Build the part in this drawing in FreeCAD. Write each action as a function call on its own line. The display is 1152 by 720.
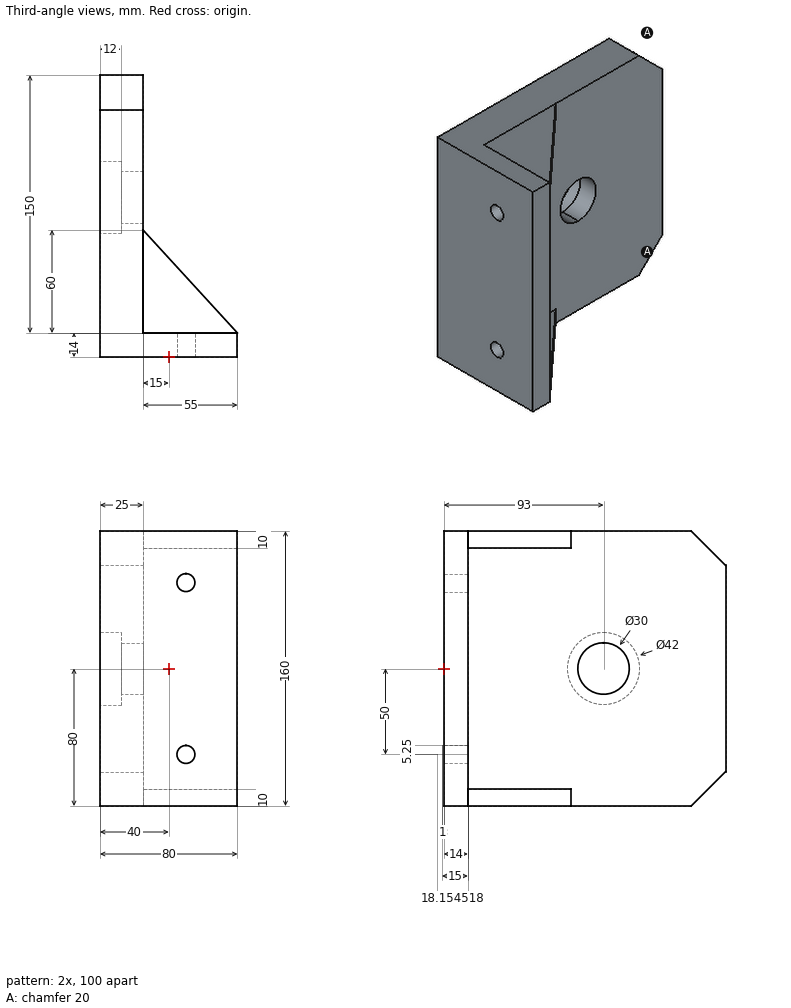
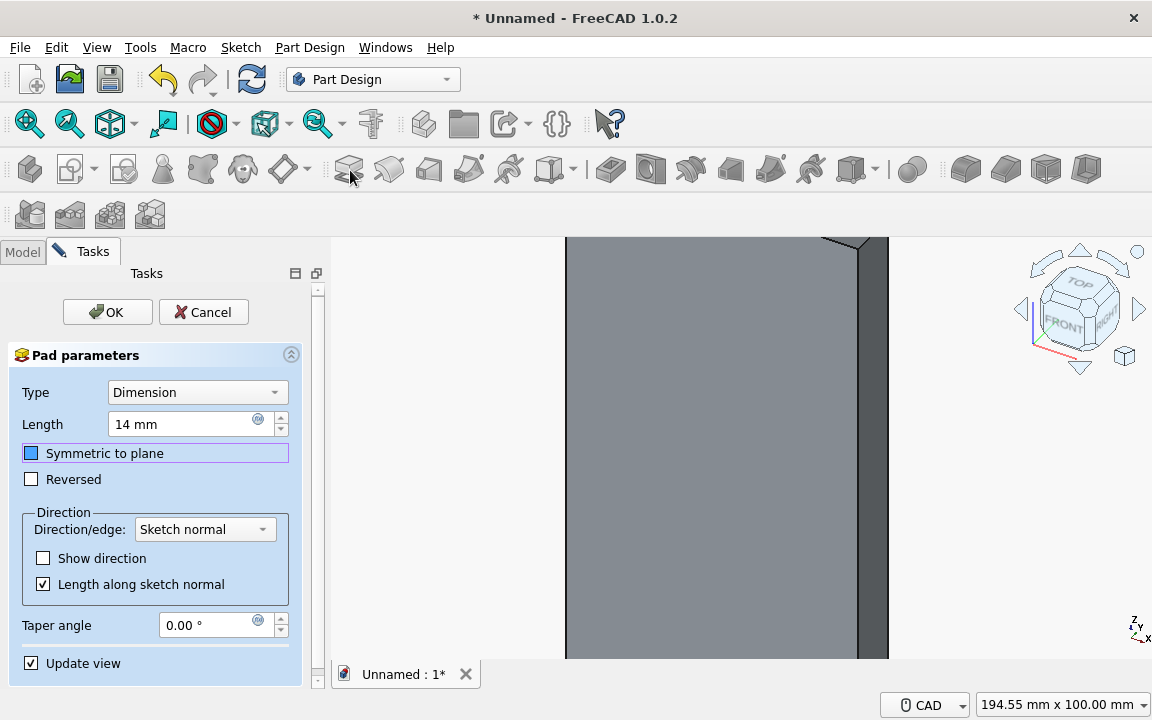
click(30, 479)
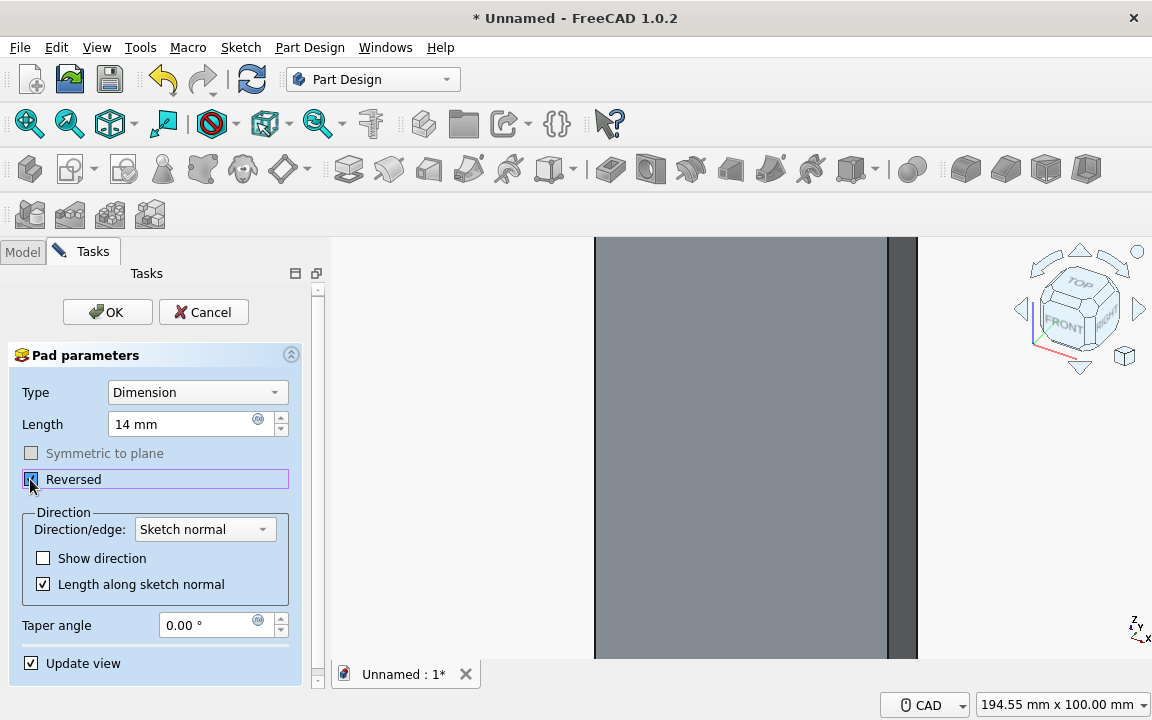
click(108, 312)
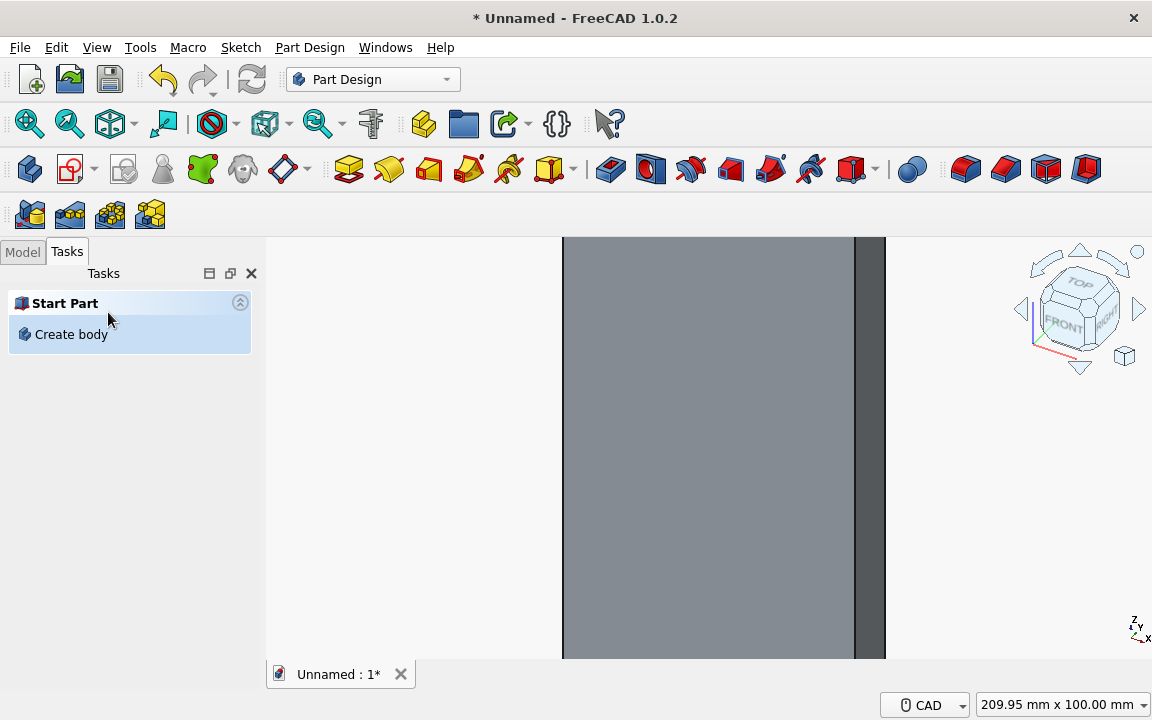
key(v)
key(f)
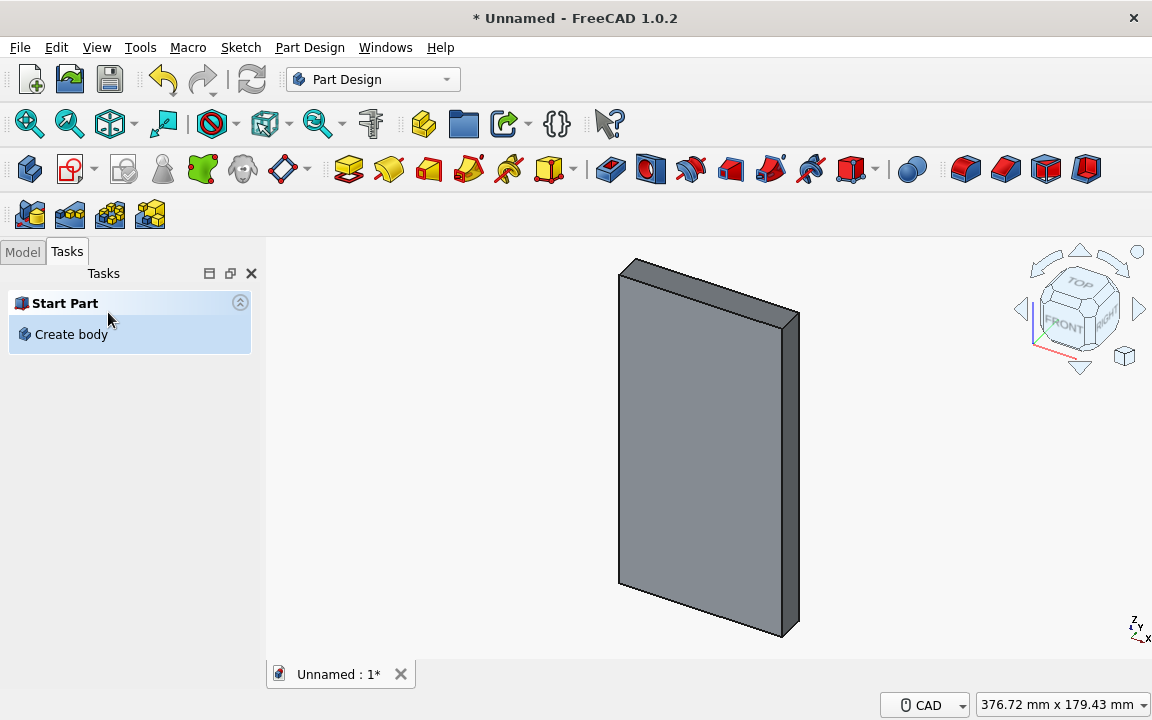
key(4)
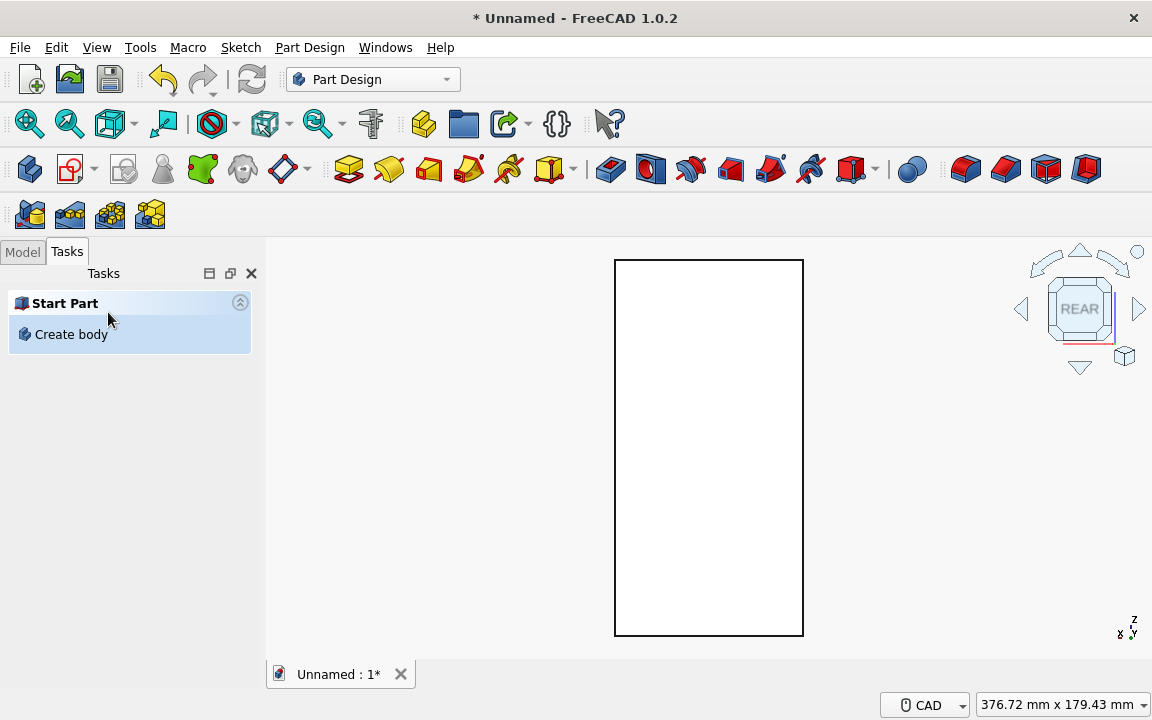
click(709, 393)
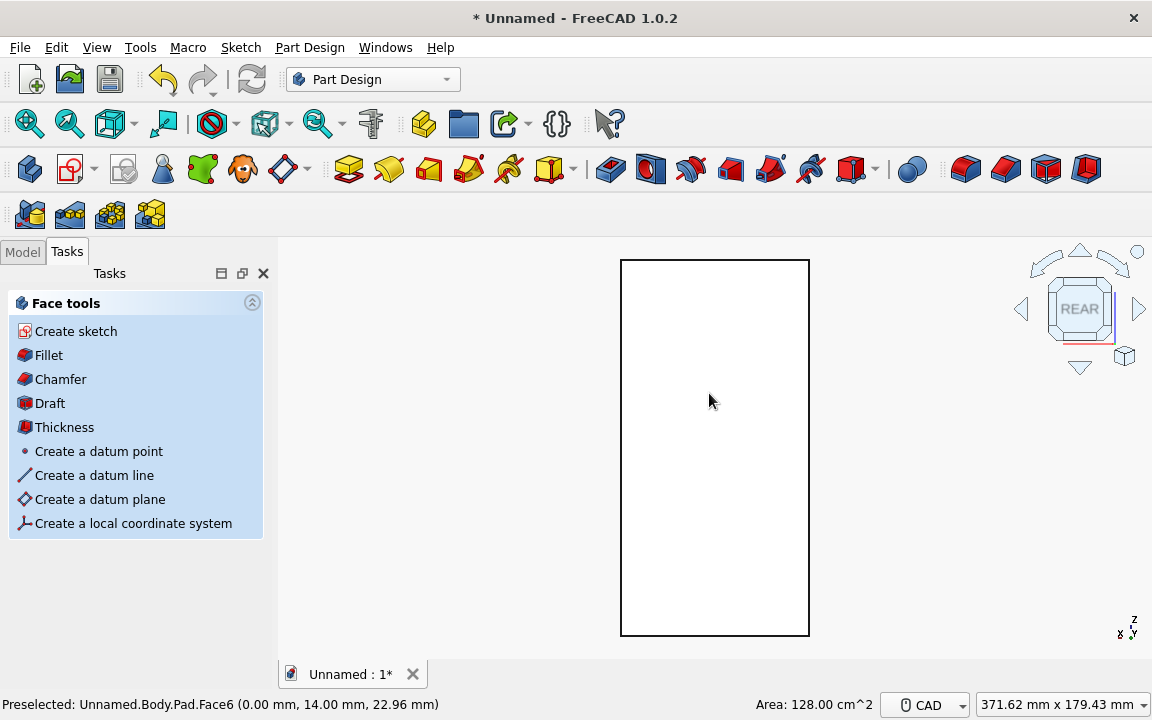
click(70, 170)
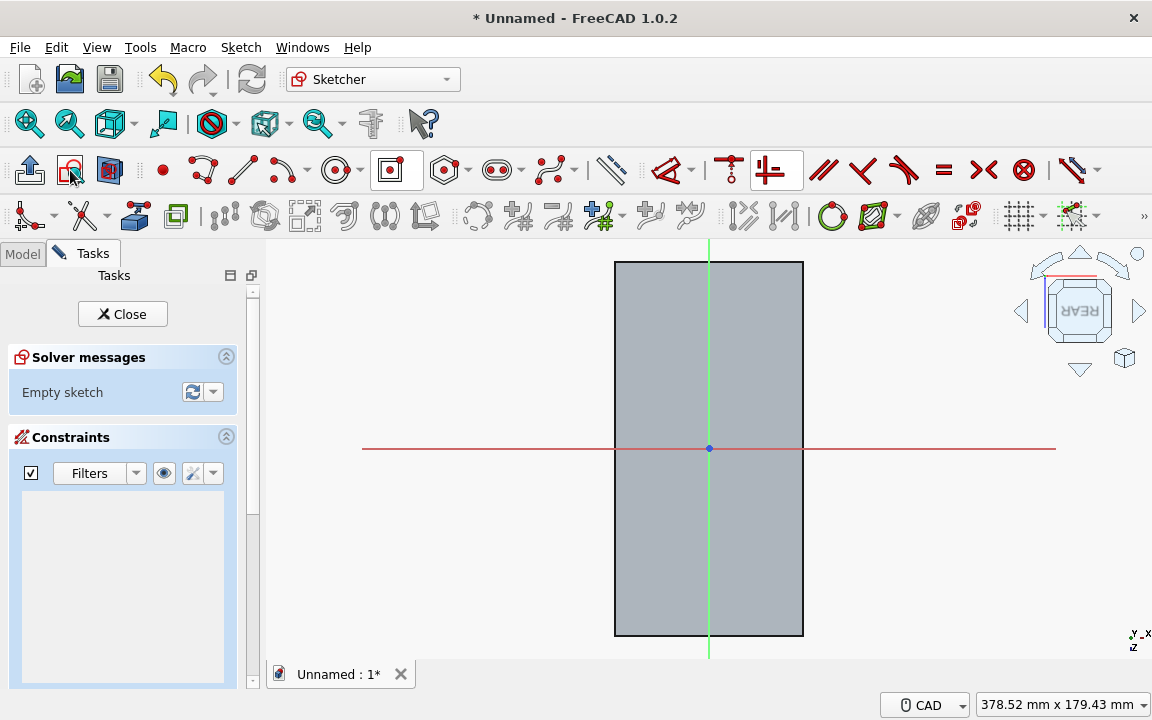
scroll(596, 449, down, 2)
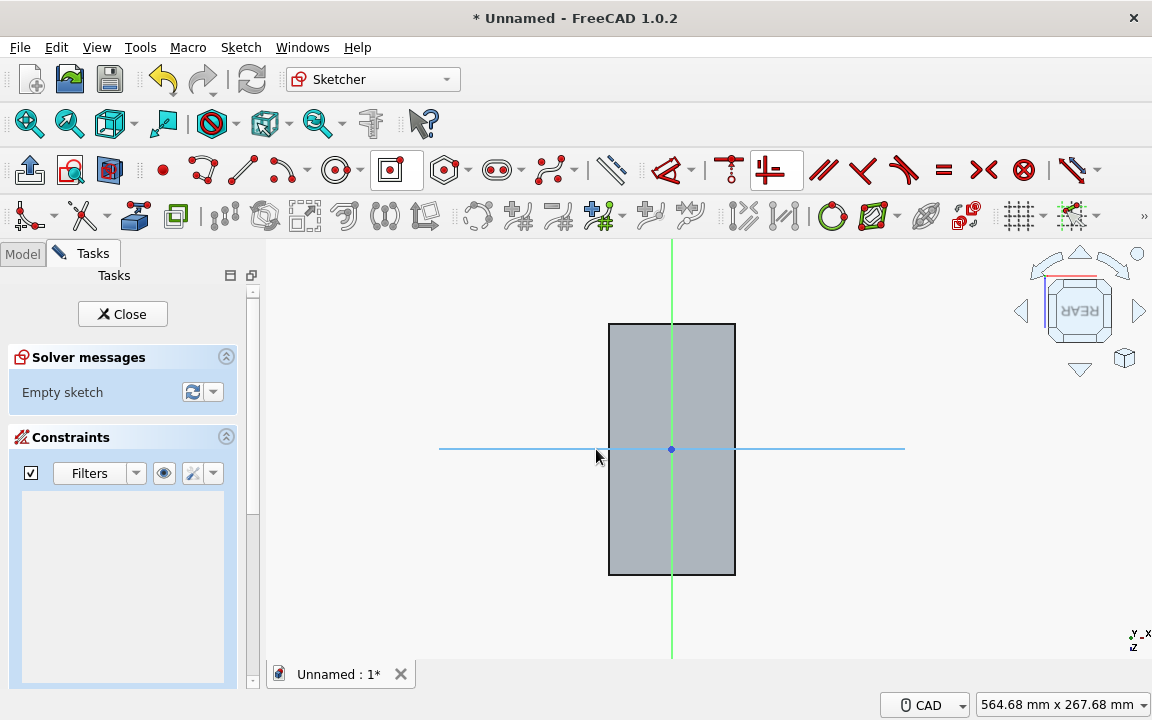
key(g)
key(r)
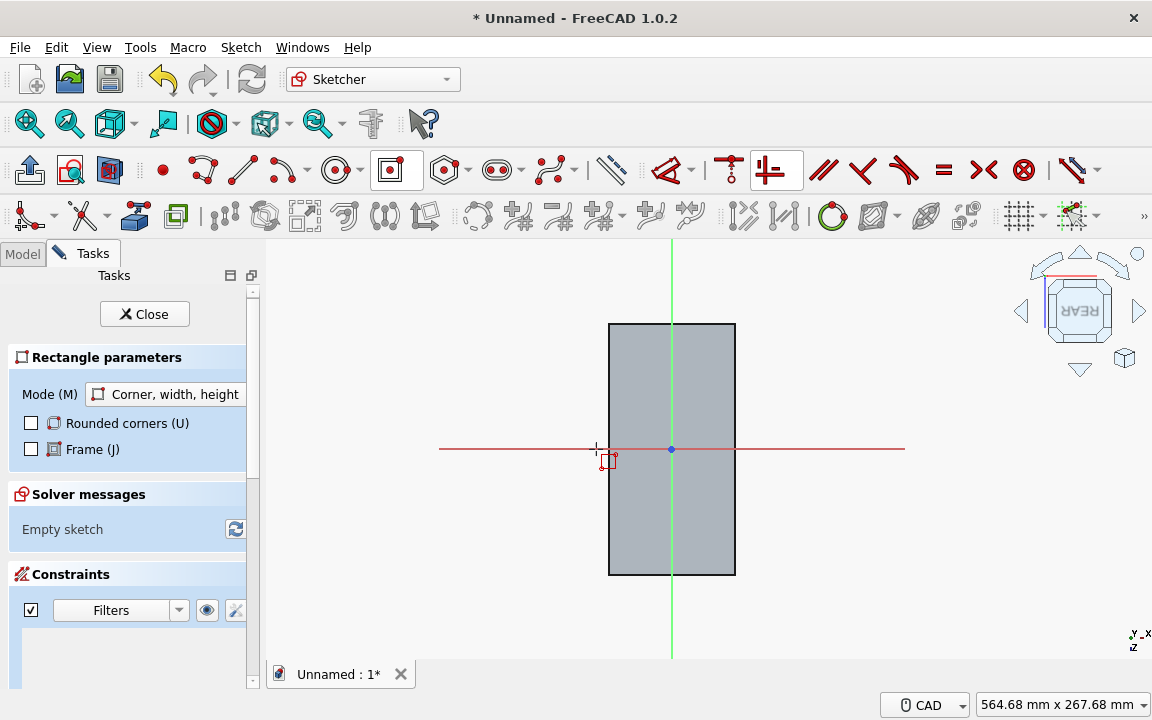
click(609, 324)
move(648, 575)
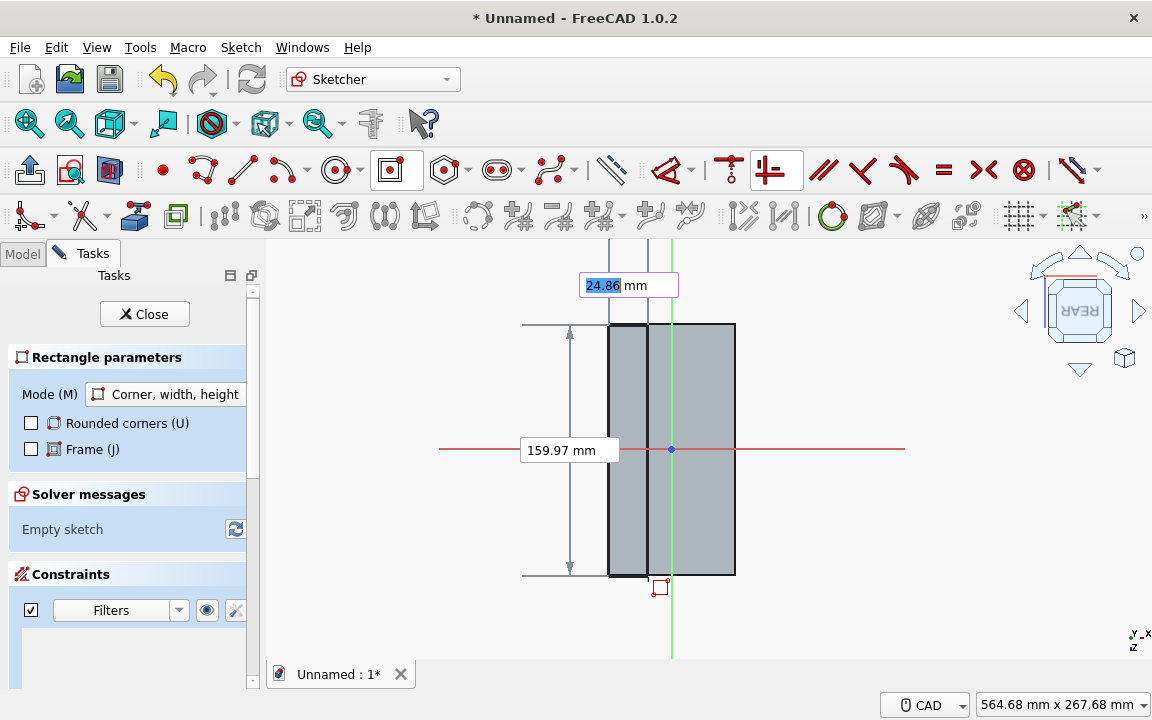
text(25)
key(Tab)
text(160)
key(Return)
key(Escape)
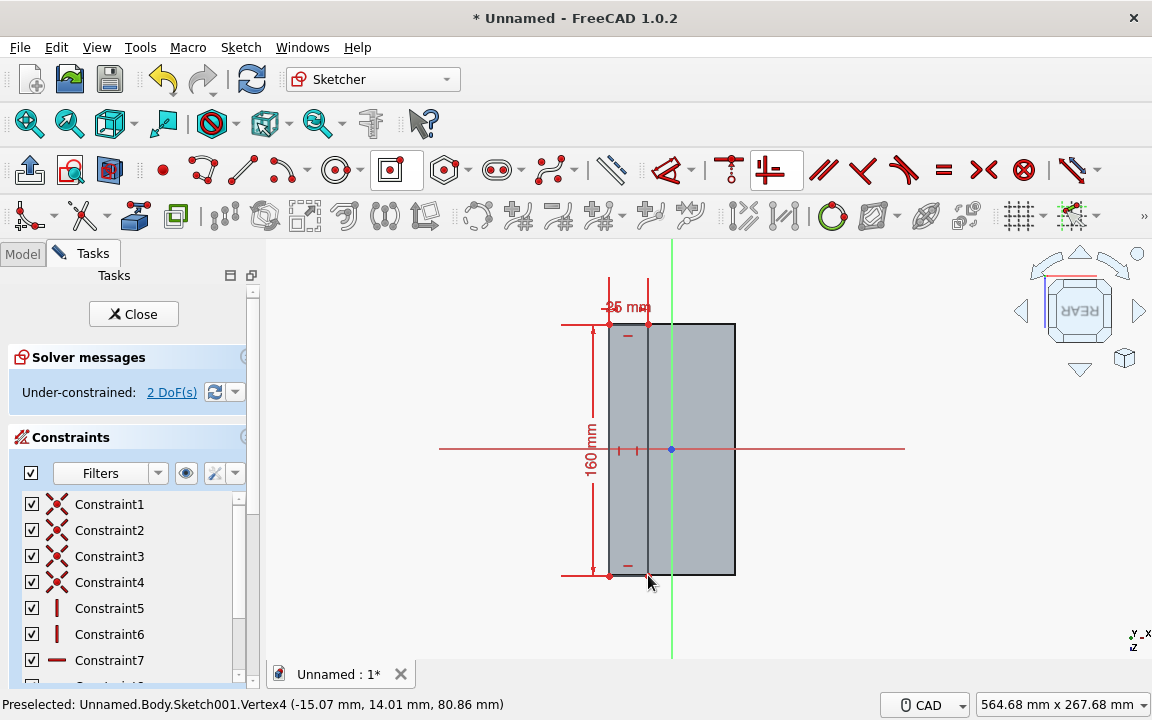
key(d)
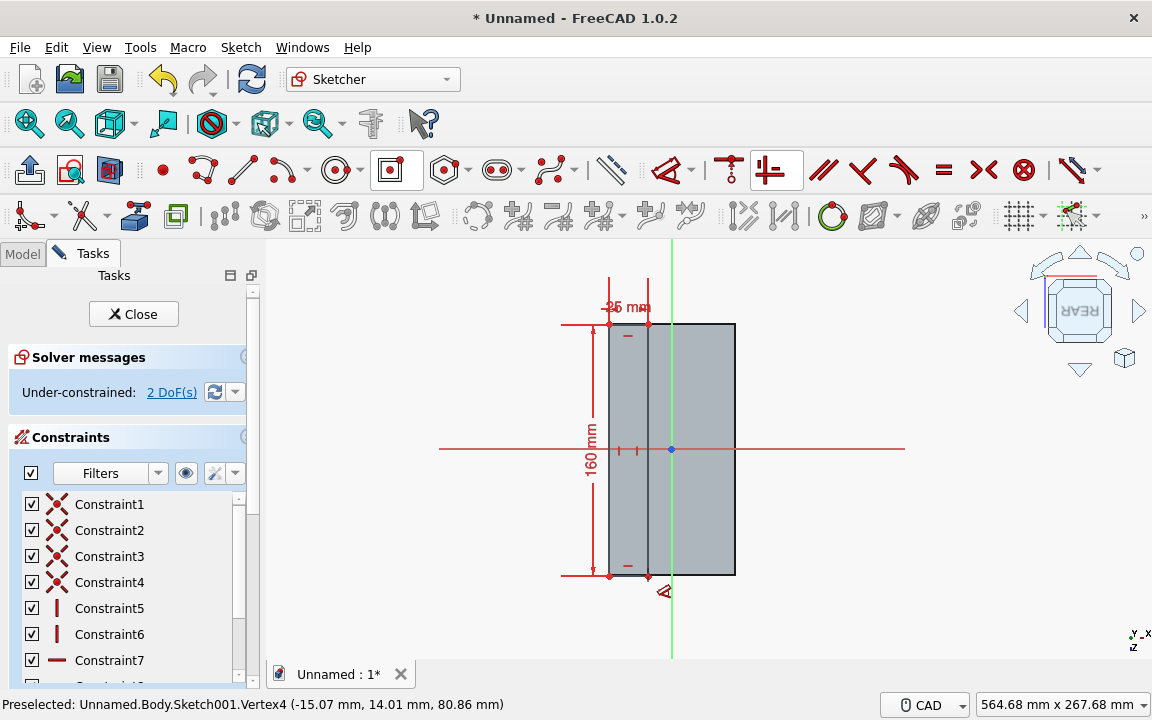
click(609, 325)
click(640, 291)